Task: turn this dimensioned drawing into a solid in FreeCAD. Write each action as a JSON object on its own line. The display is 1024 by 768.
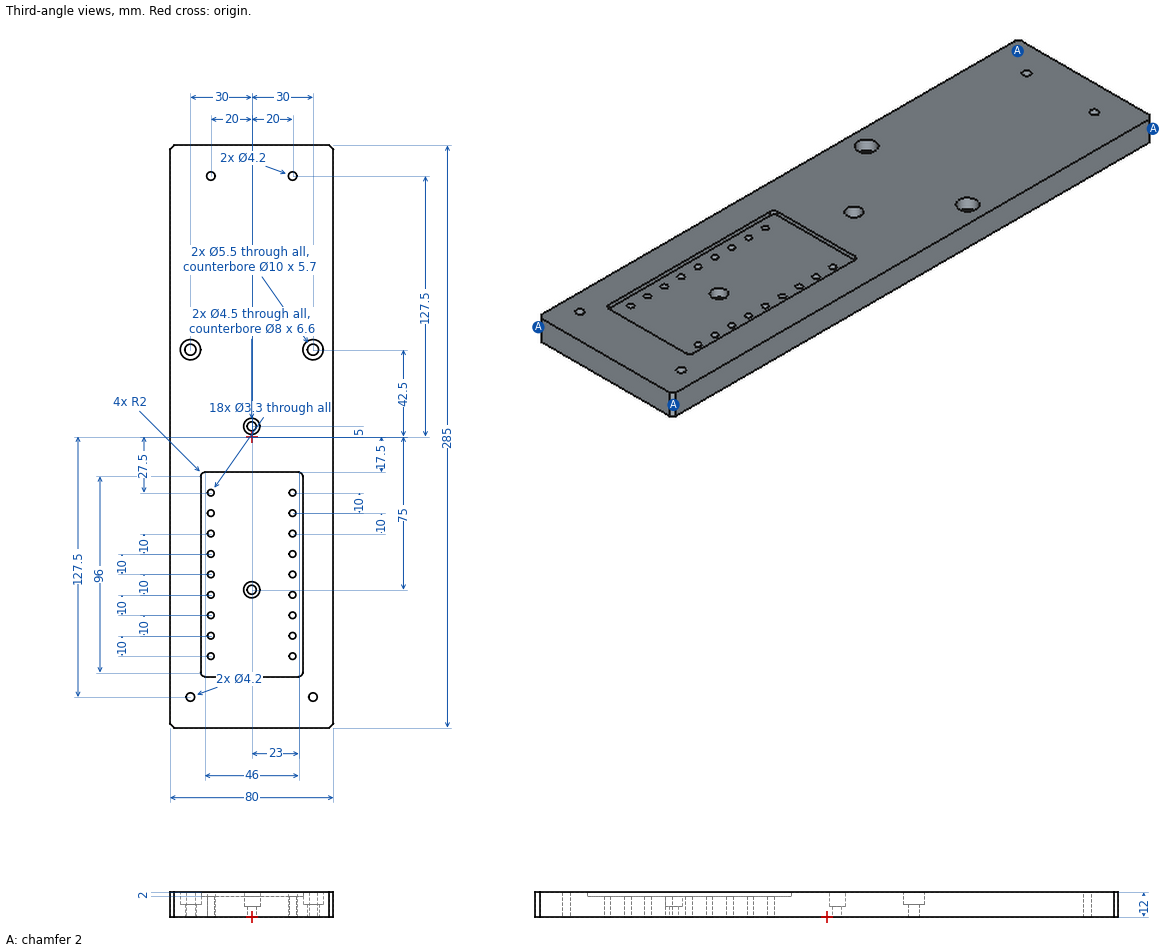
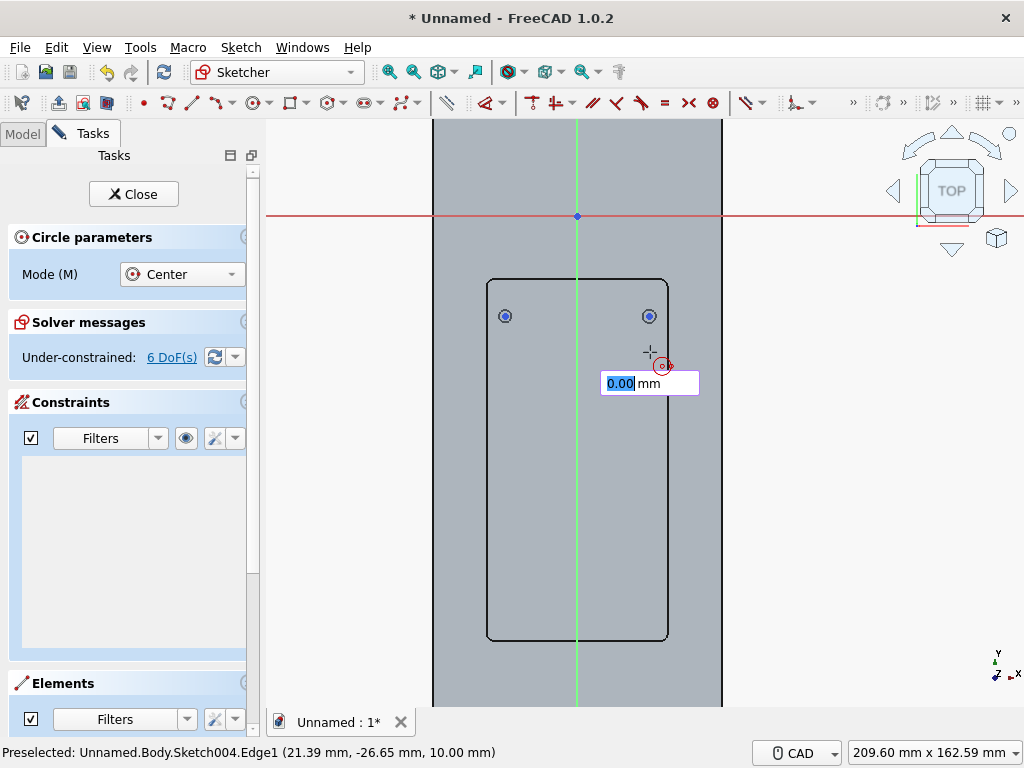
{"action": "scroll", "coordinate": [654, 347], "scroll_direction": "up", "scroll_amount": 5}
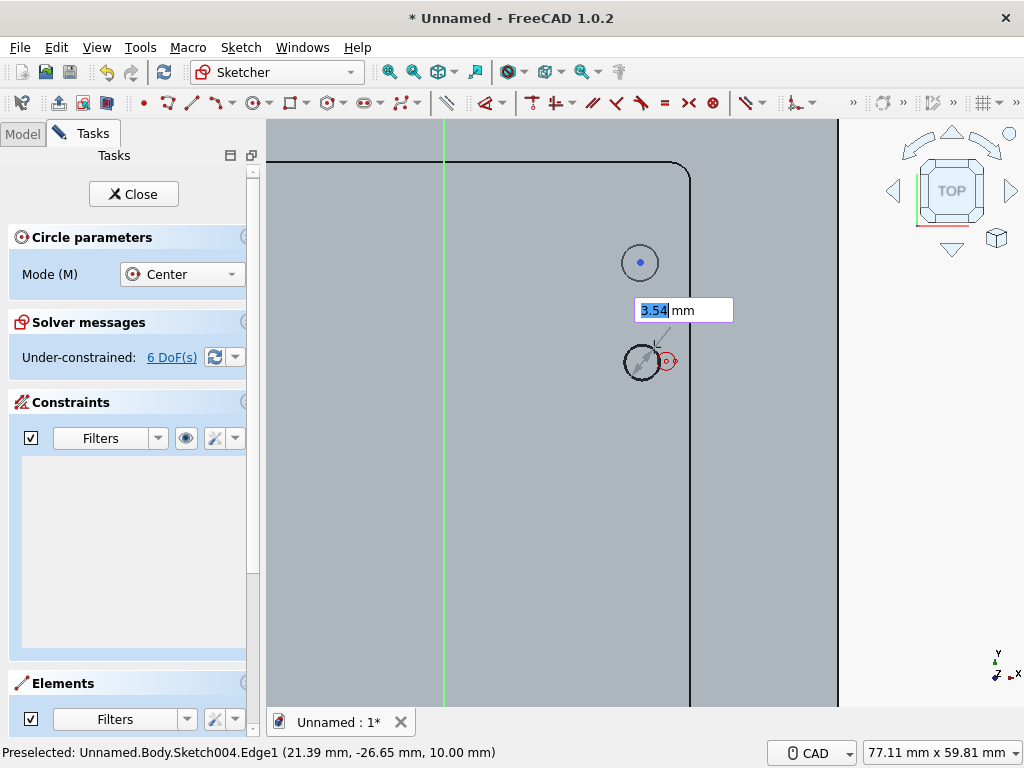
{"action": "left_click", "coordinate": [652, 348]}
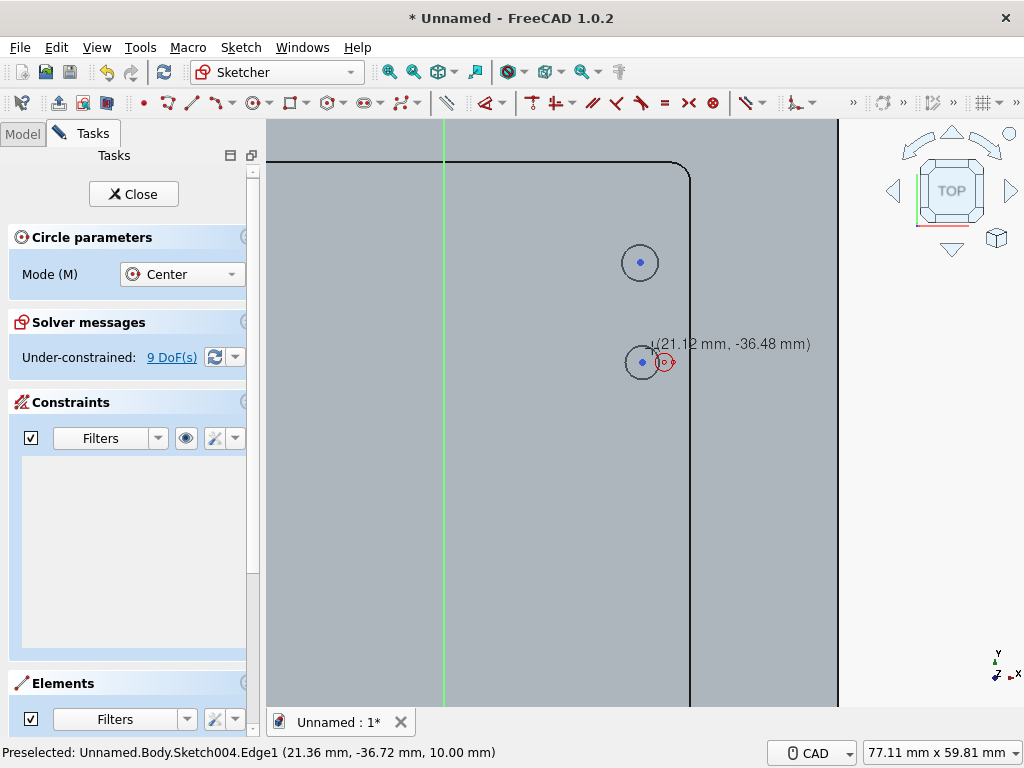
{"action": "scroll", "coordinate": [641, 457], "scroll_direction": "up", "scroll_amount": 2}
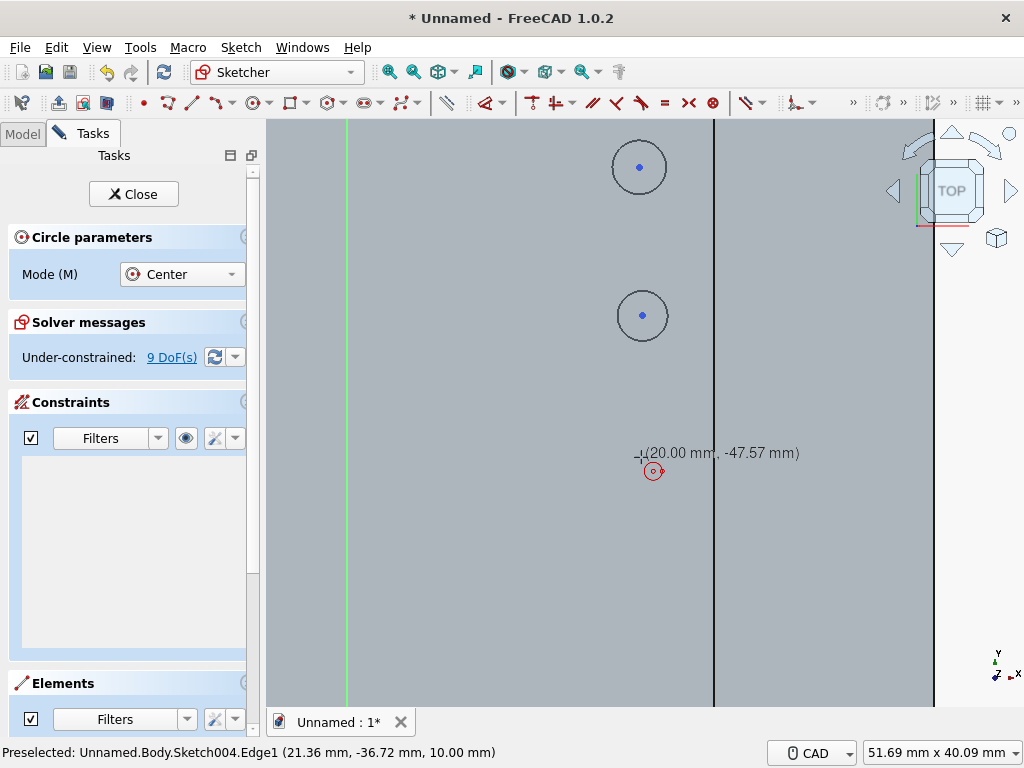
{"action": "scroll", "coordinate": [651, 365], "scroll_direction": "down", "scroll_amount": 7}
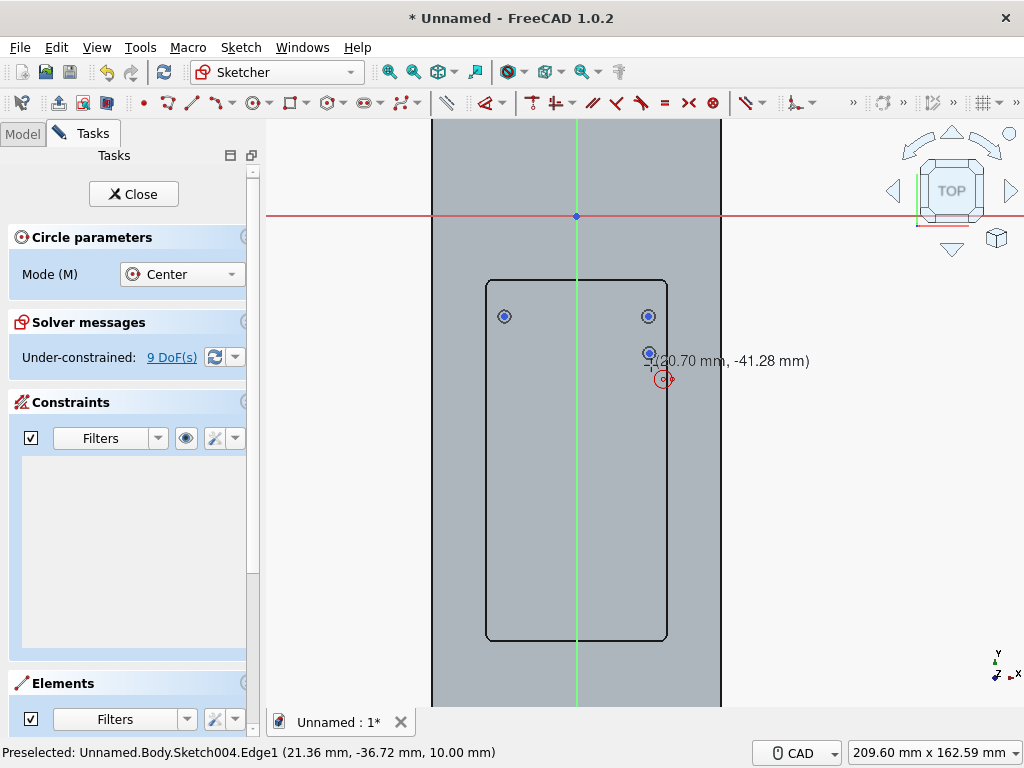
{"action": "left_click", "coordinate": [649, 388]}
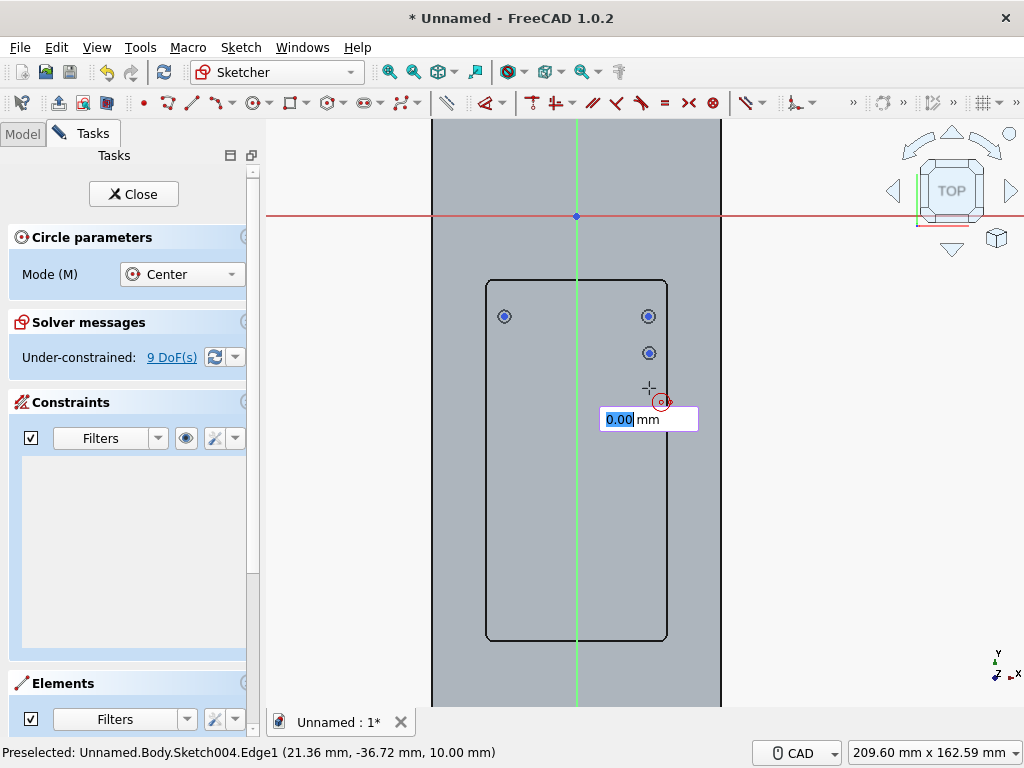
{"action": "scroll", "coordinate": [653, 384], "scroll_direction": "up", "scroll_amount": 5}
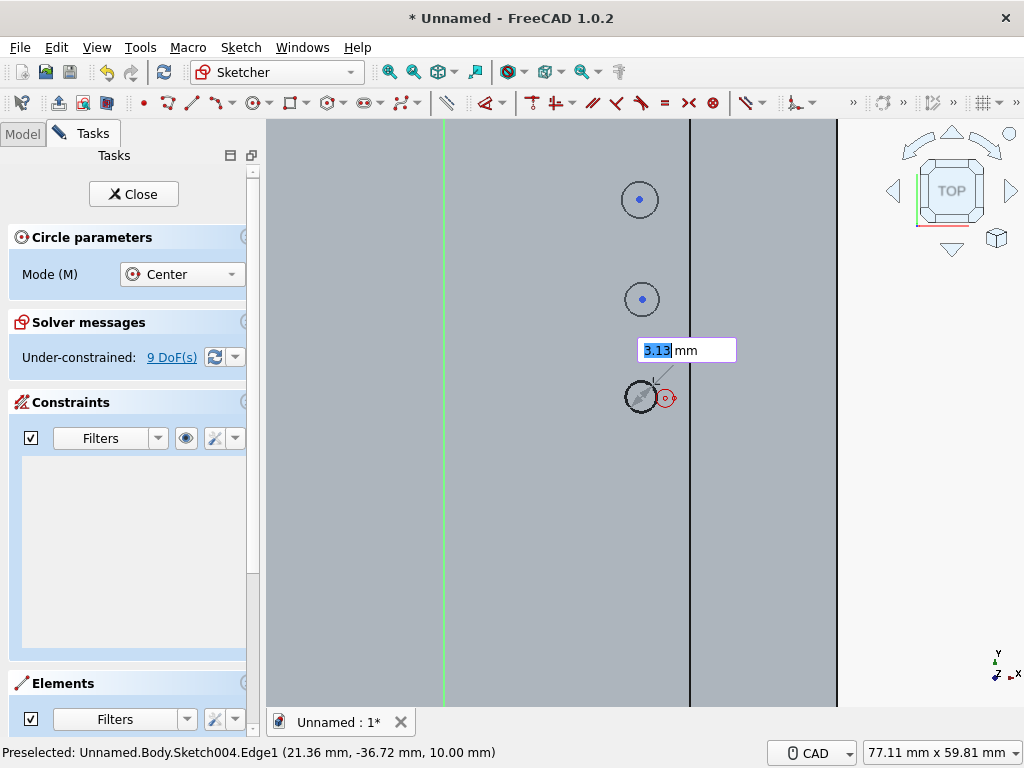
{"action": "left_click", "coordinate": [652, 383]}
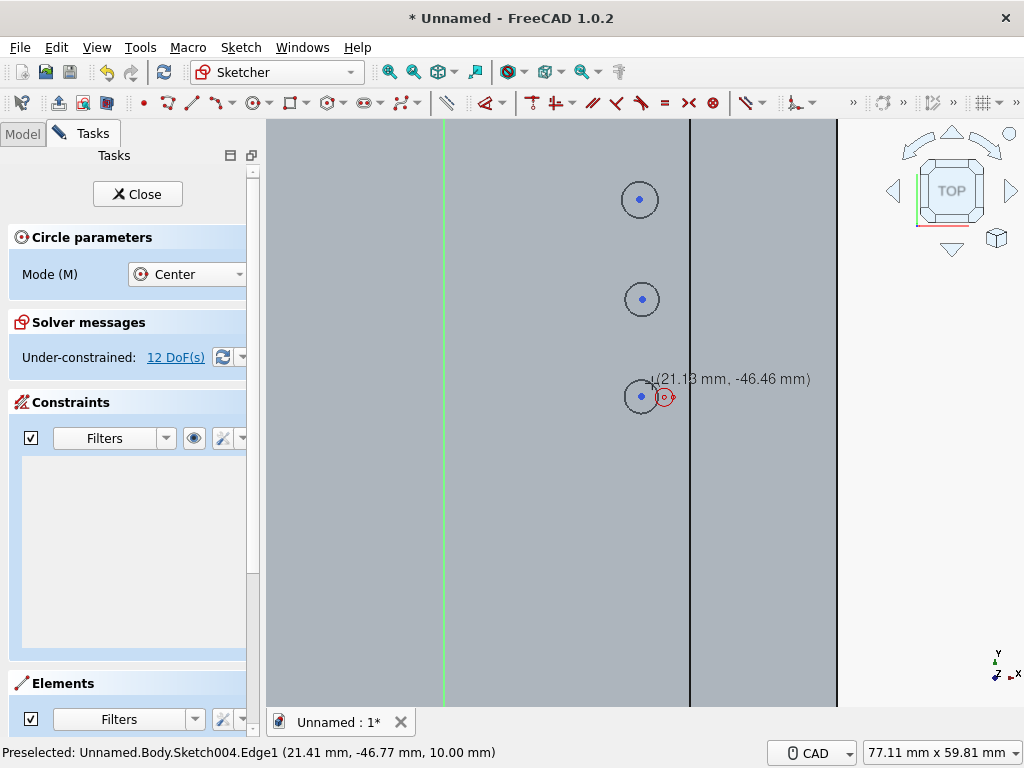
{"action": "scroll", "coordinate": [653, 383], "scroll_direction": "down", "scroll_amount": 5}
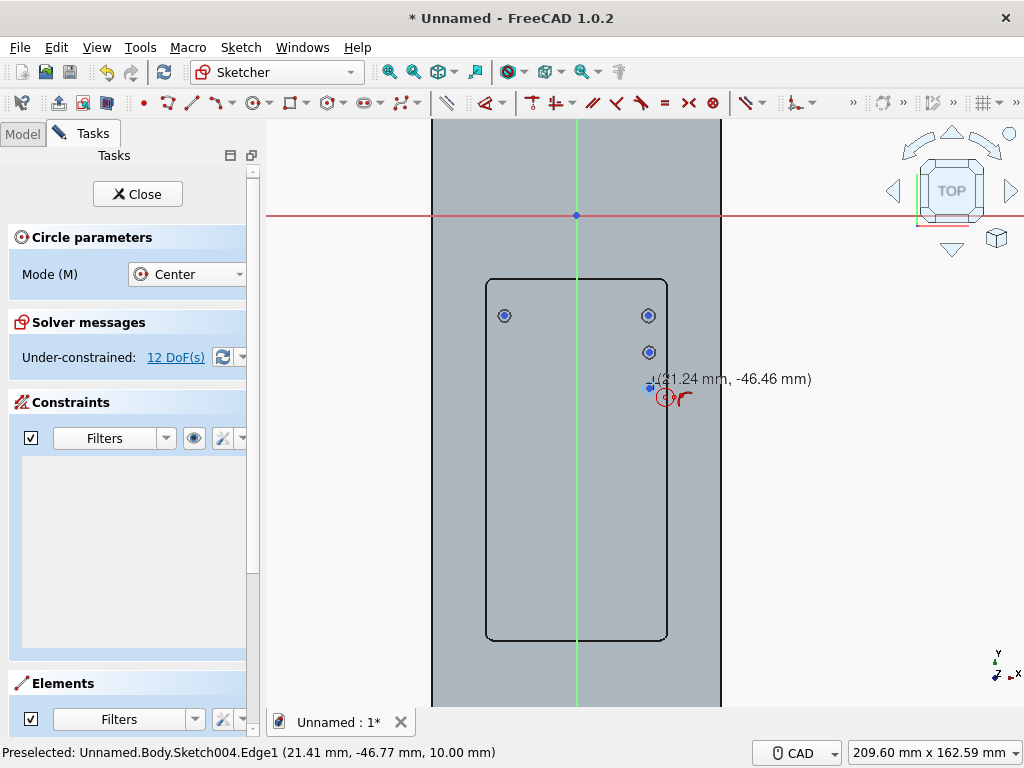
{"action": "scroll", "coordinate": [504, 351], "scroll_direction": "up", "scroll_amount": 7}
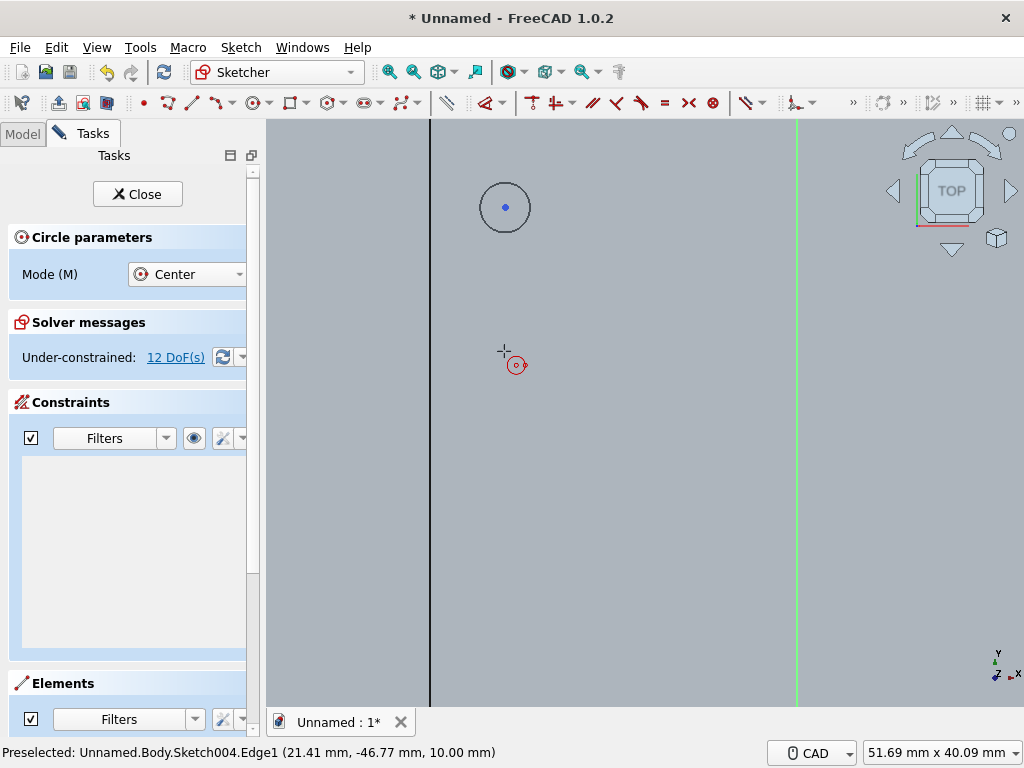
{"action": "scroll", "coordinate": [504, 351], "scroll_direction": "down", "scroll_amount": 7}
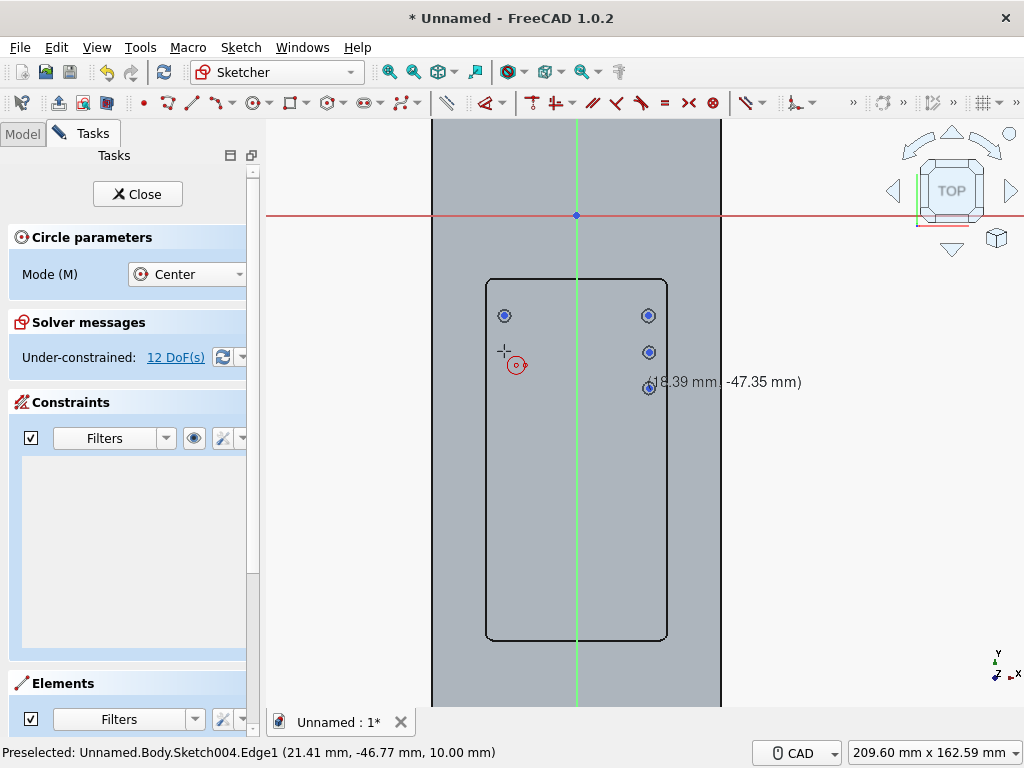
{"action": "left_click", "coordinate": [504, 351]}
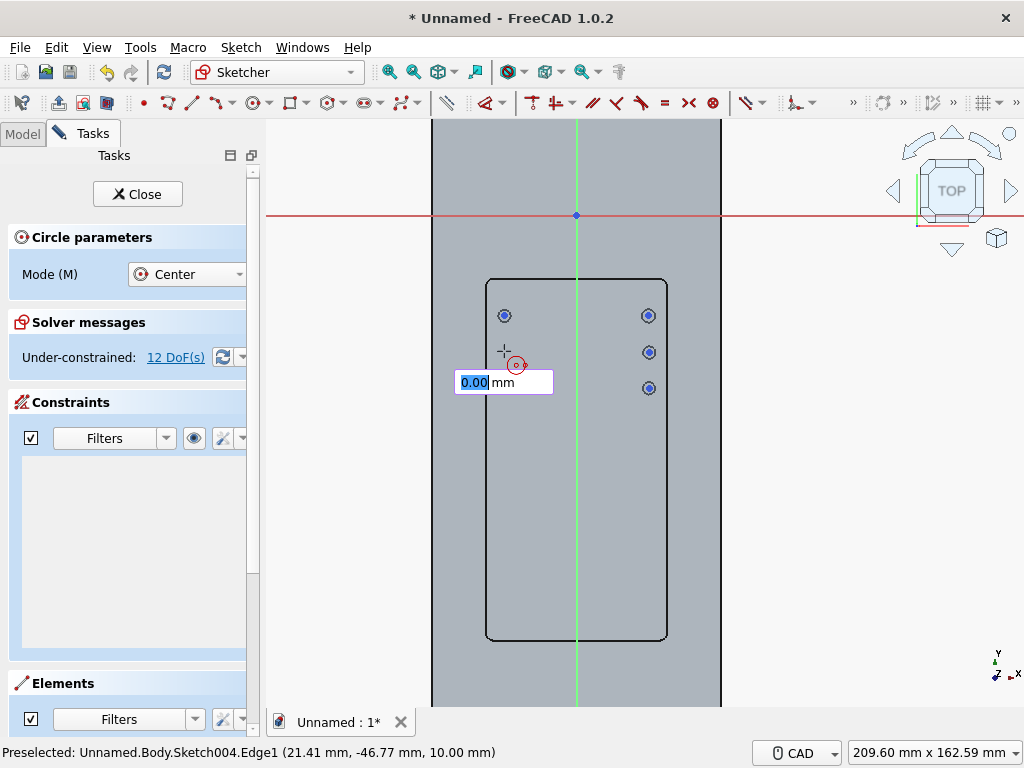
{"action": "scroll", "coordinate": [508, 347], "scroll_direction": "up", "scroll_amount": 5}